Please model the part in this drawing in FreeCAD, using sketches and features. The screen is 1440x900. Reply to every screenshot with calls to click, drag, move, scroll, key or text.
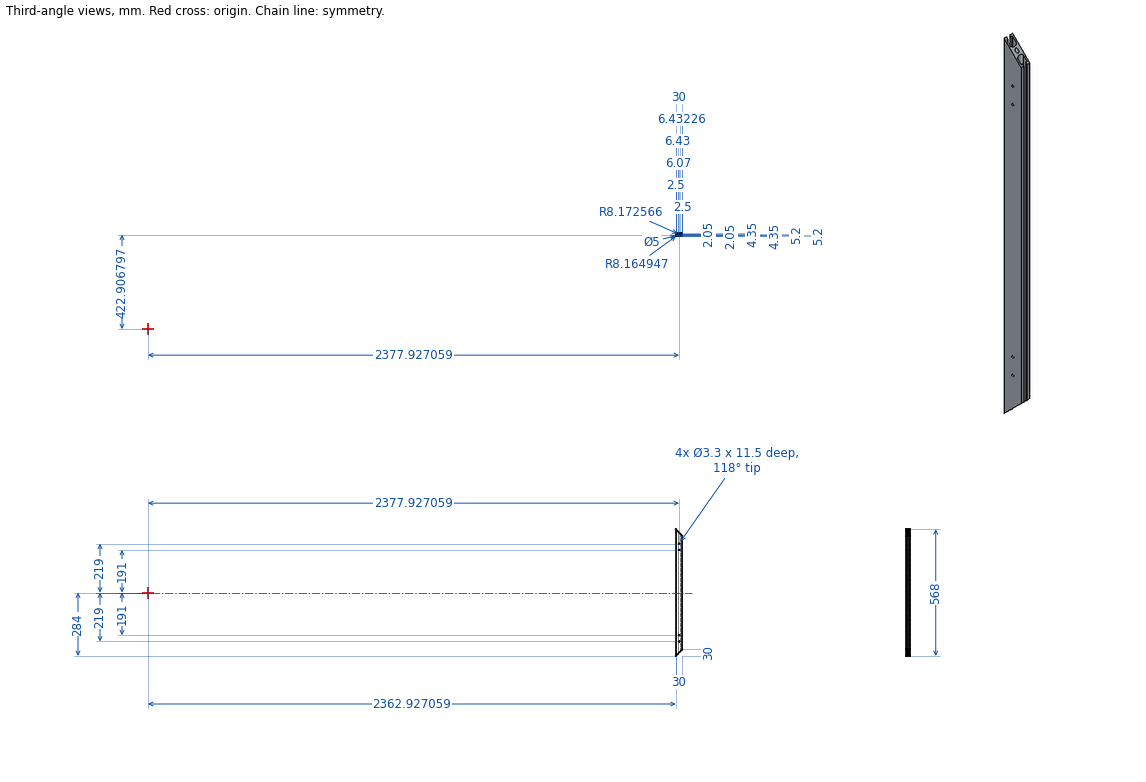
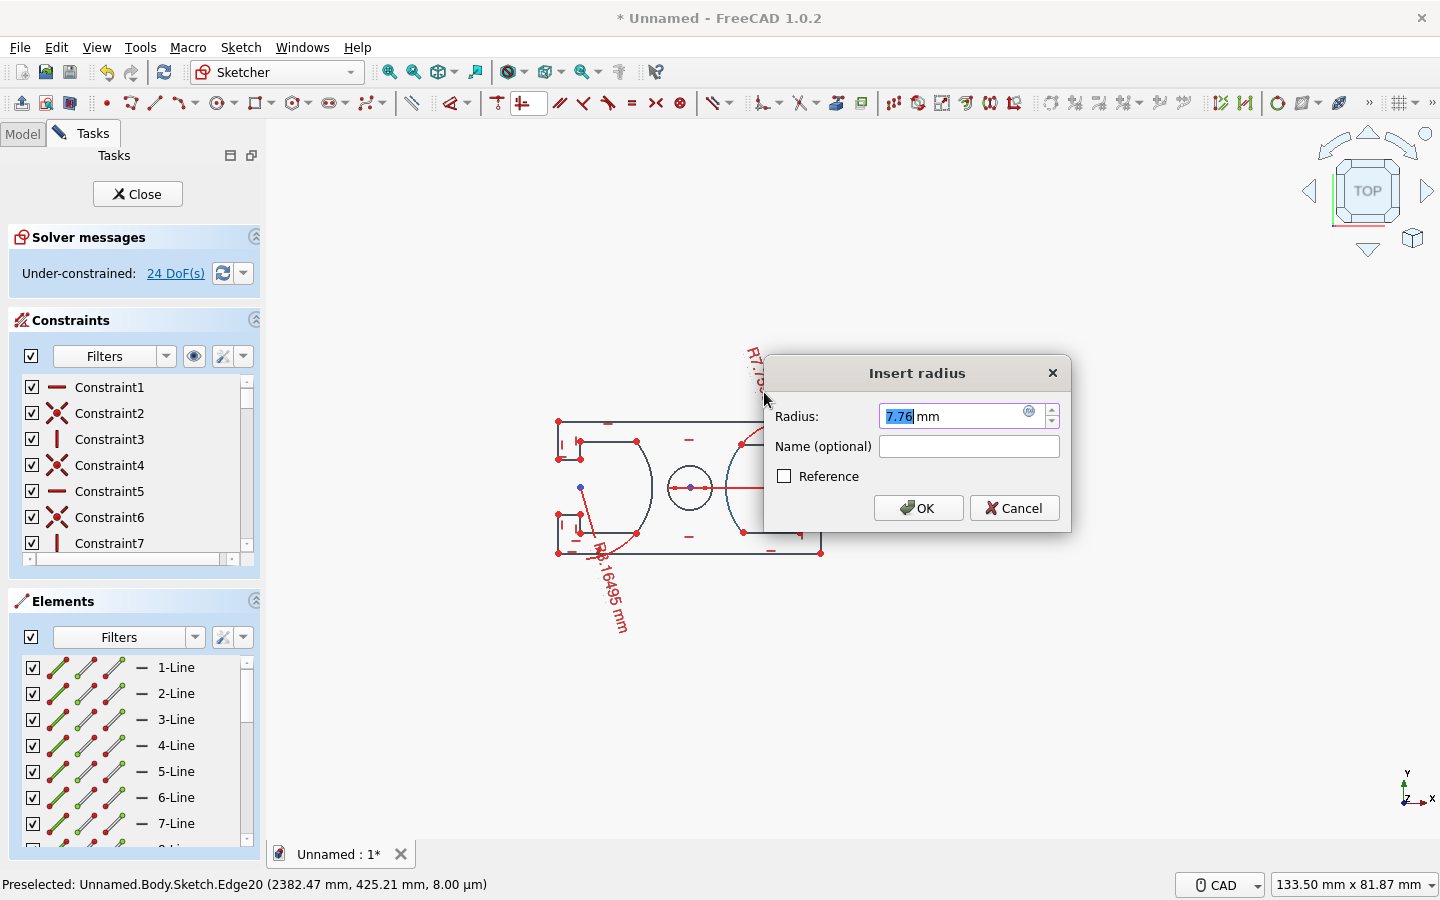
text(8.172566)
key(Return)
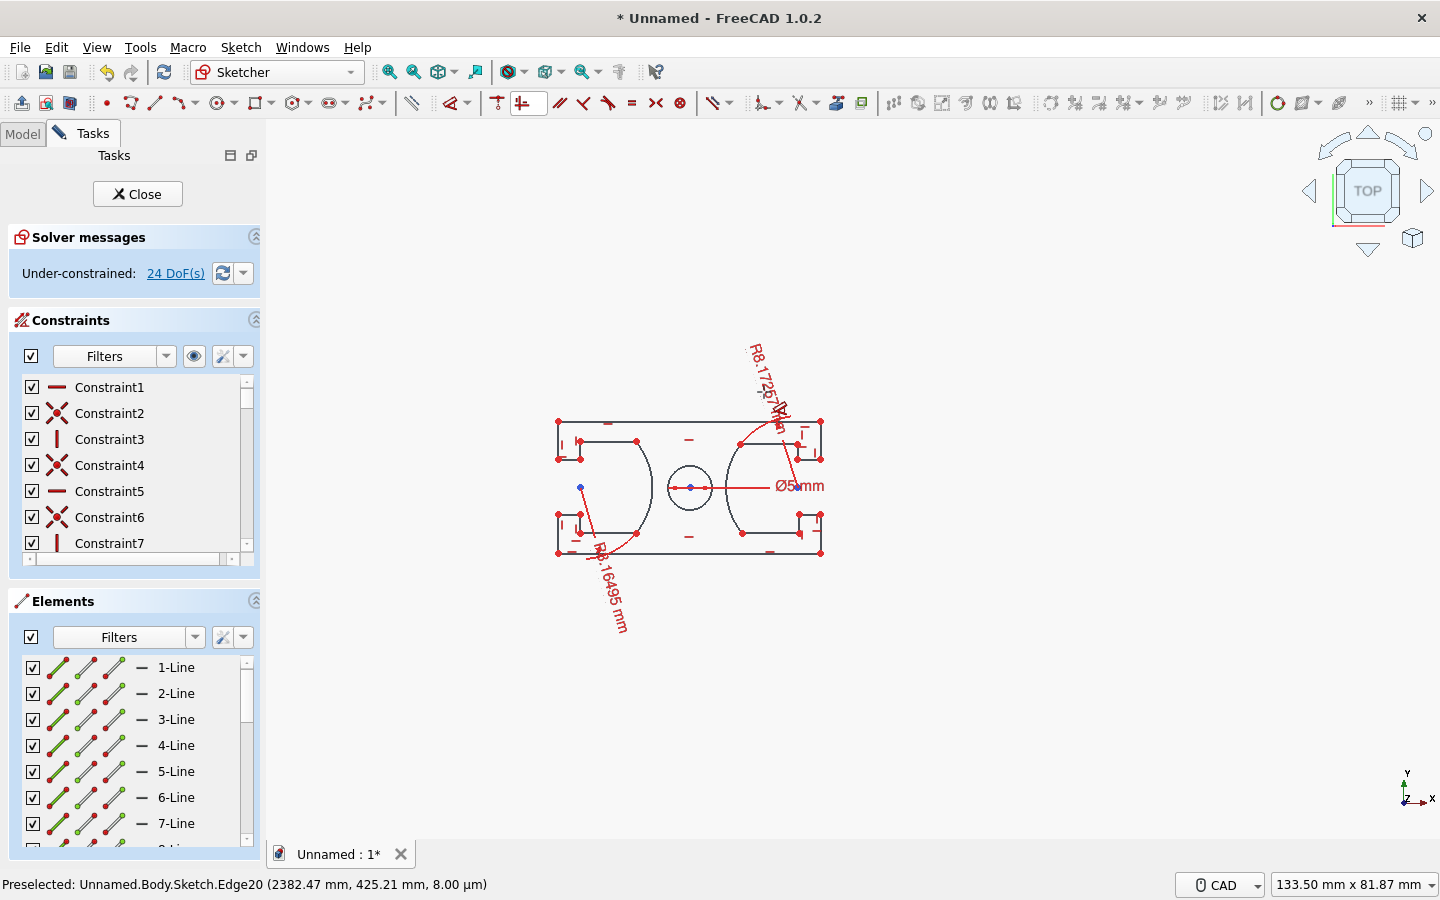
click(742, 422)
click(689, 388)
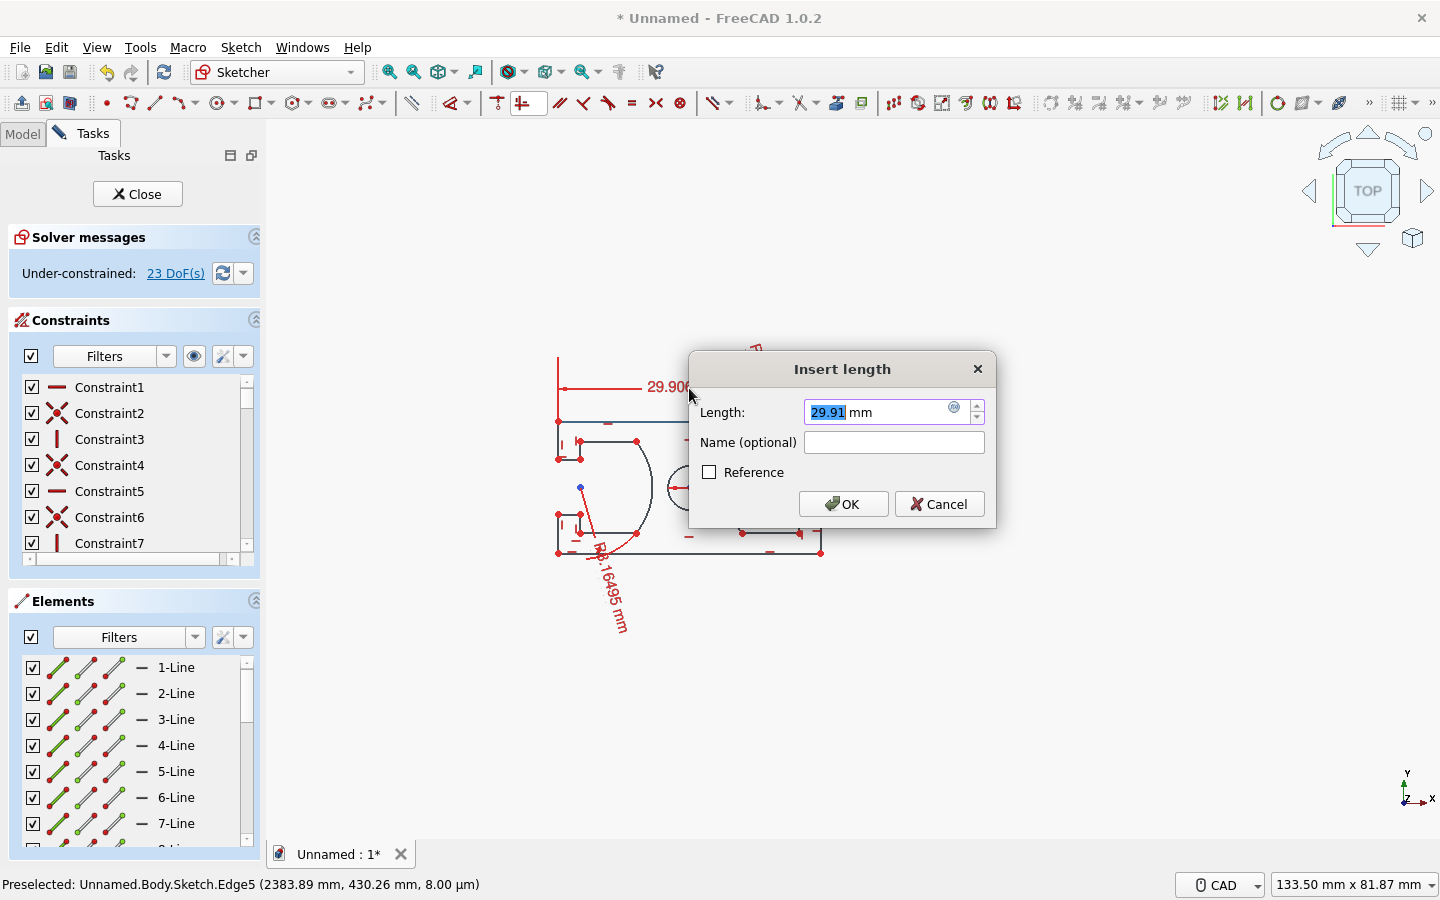
text(30)
key(Return)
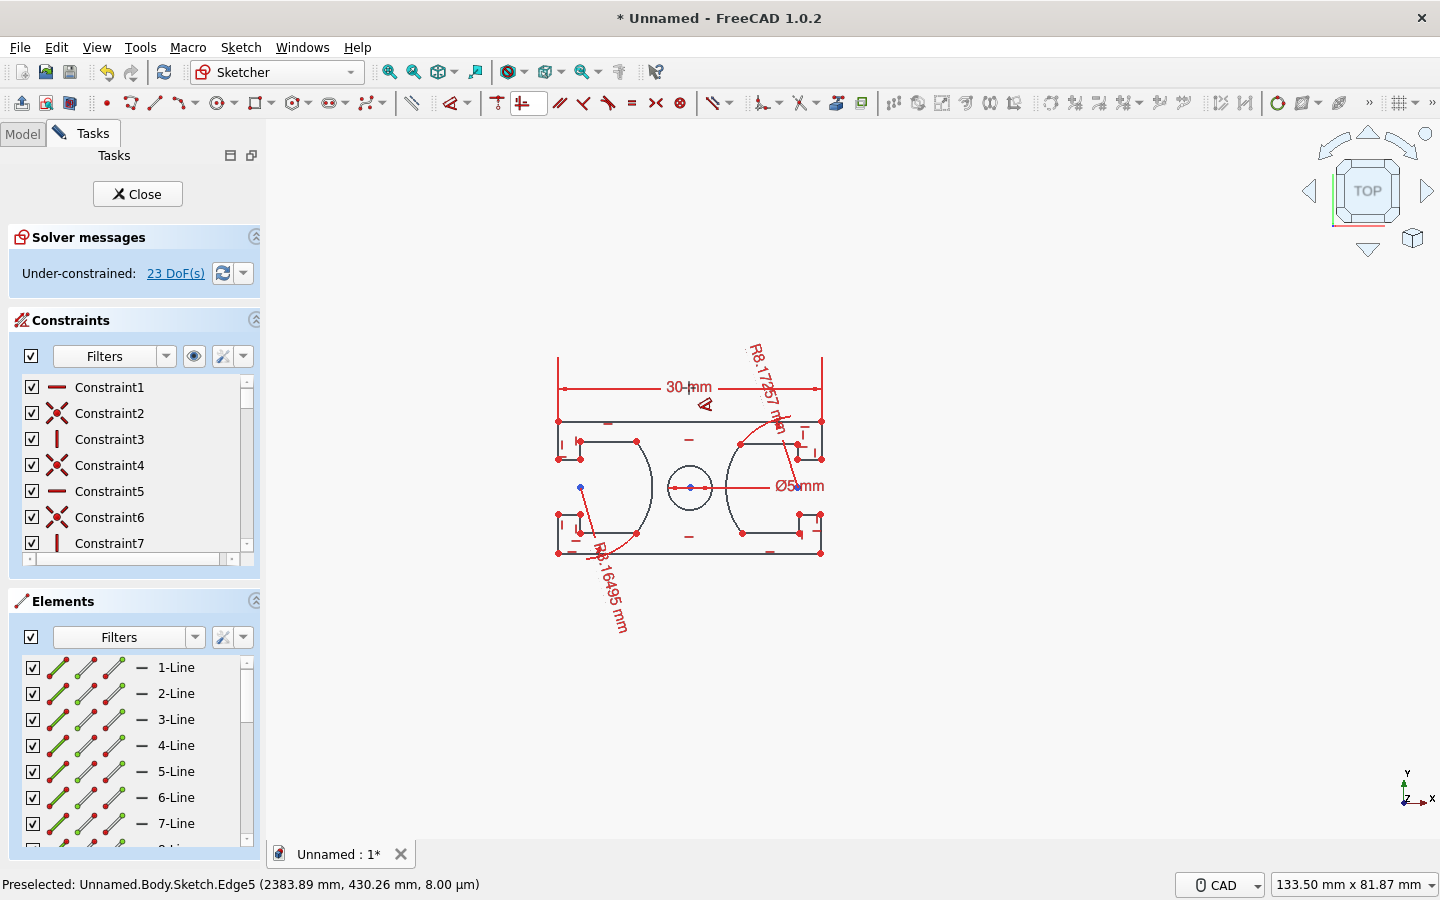
click(637, 554)
click(689, 588)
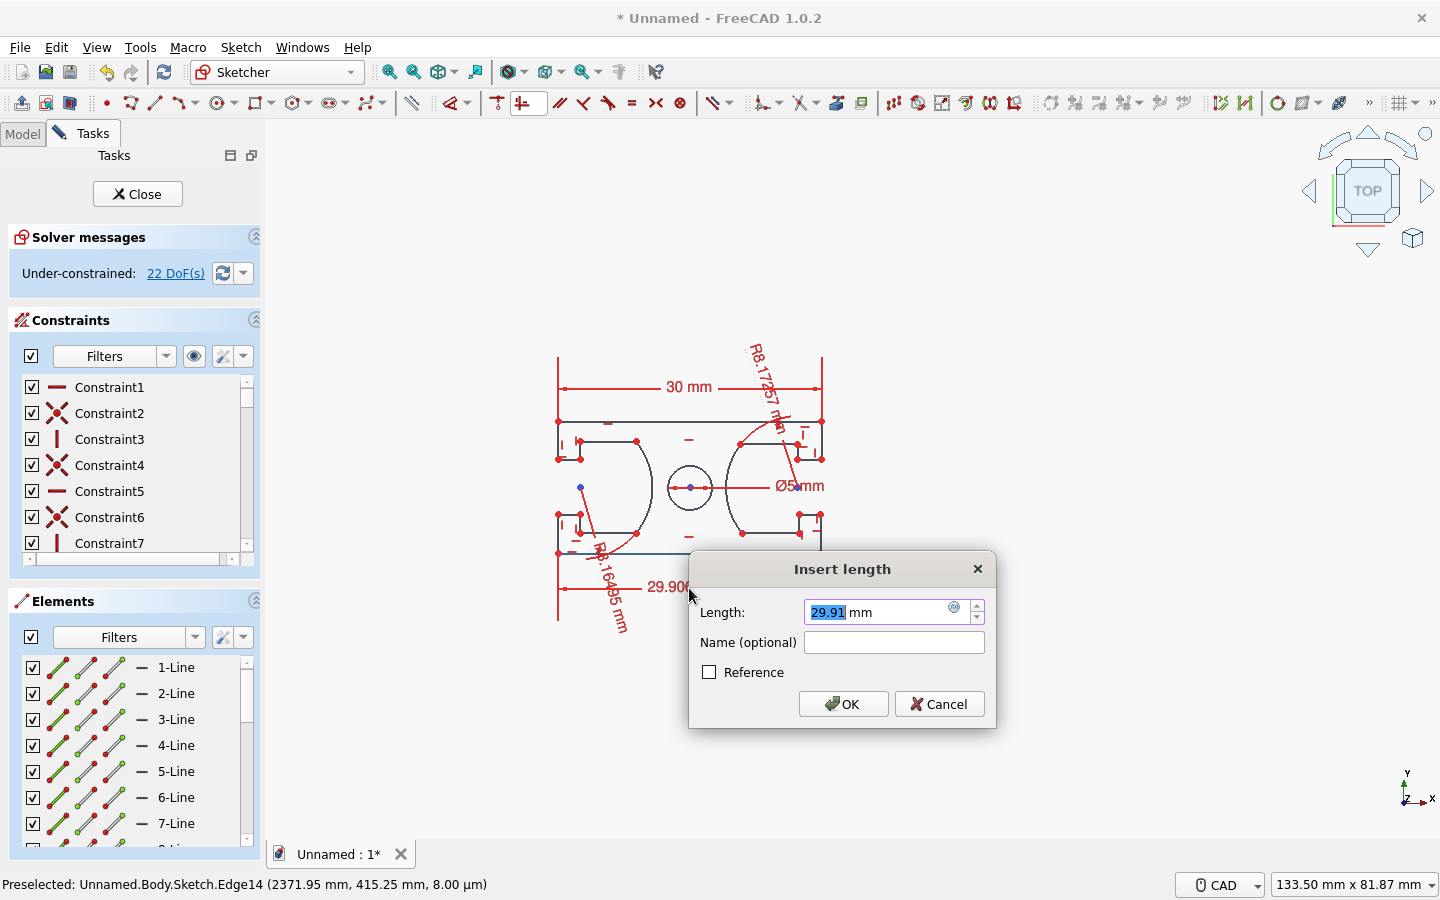
text(30)
key(Return)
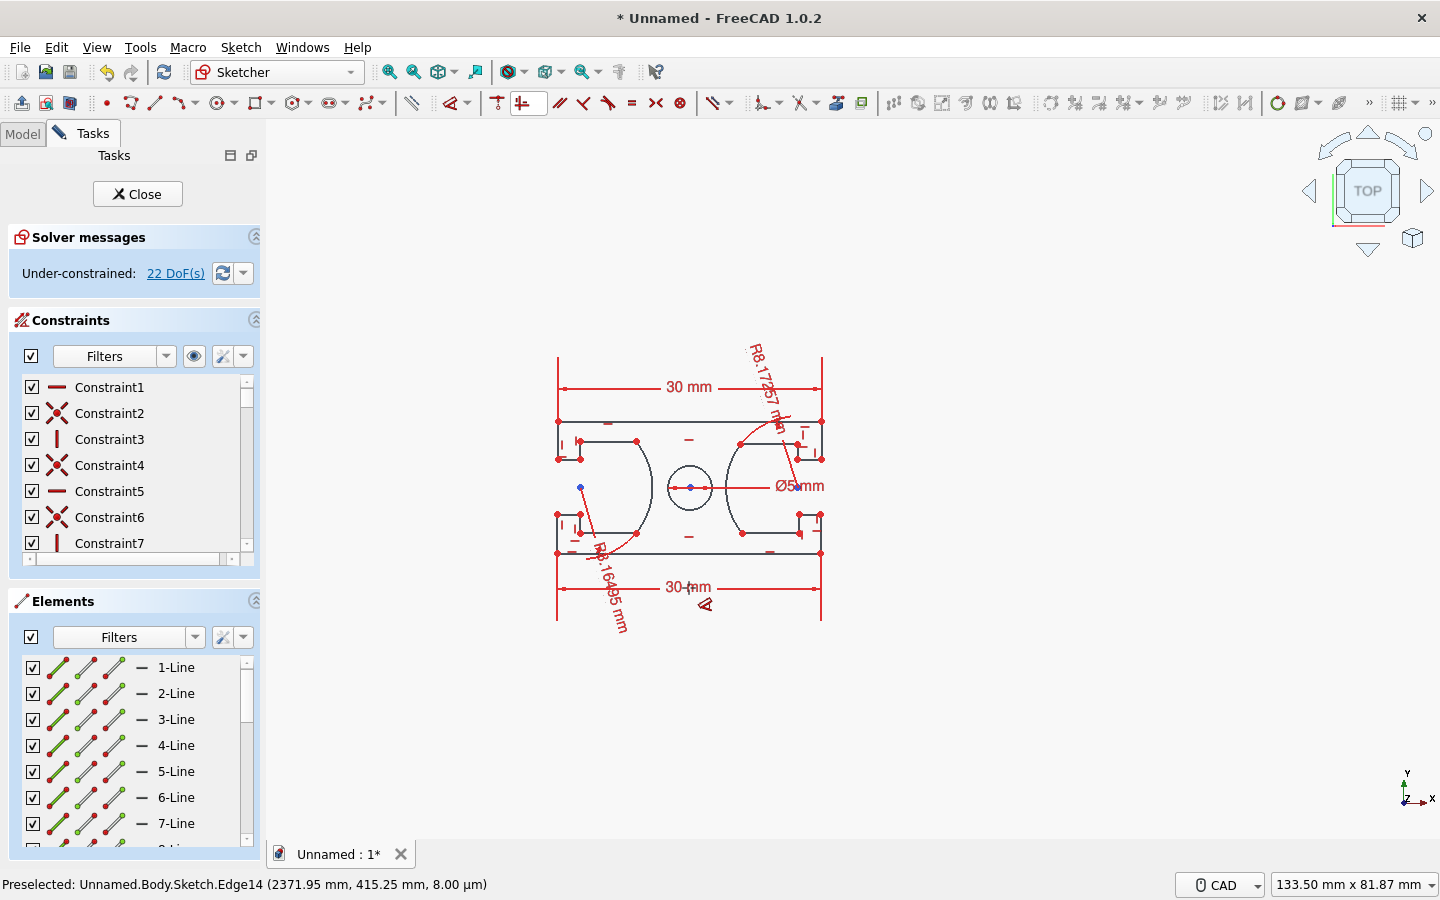
scroll(807, 460, up, 3)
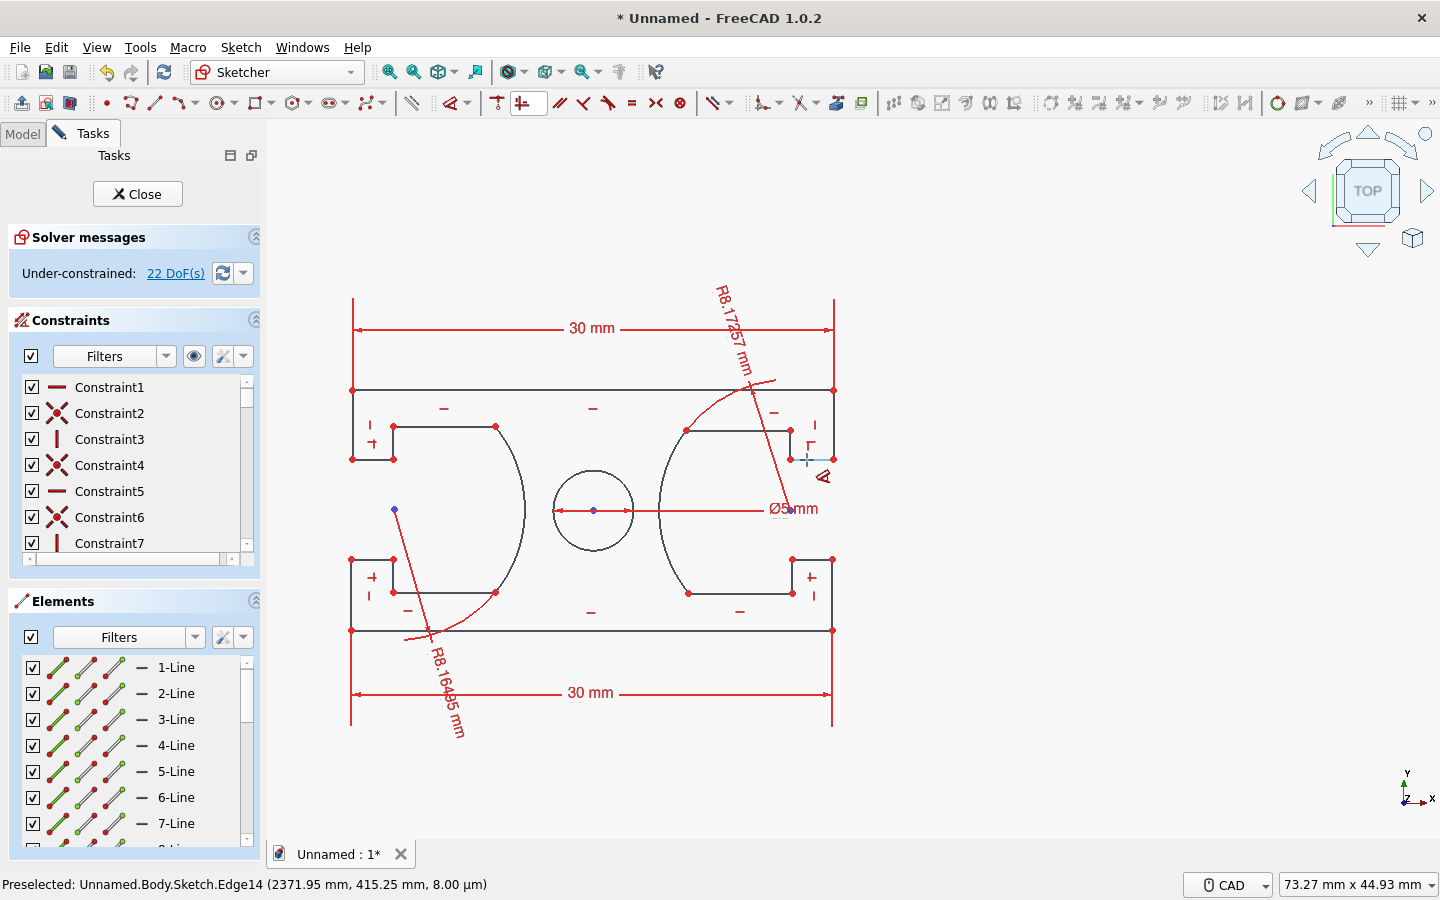
click(808, 460)
click(812, 426)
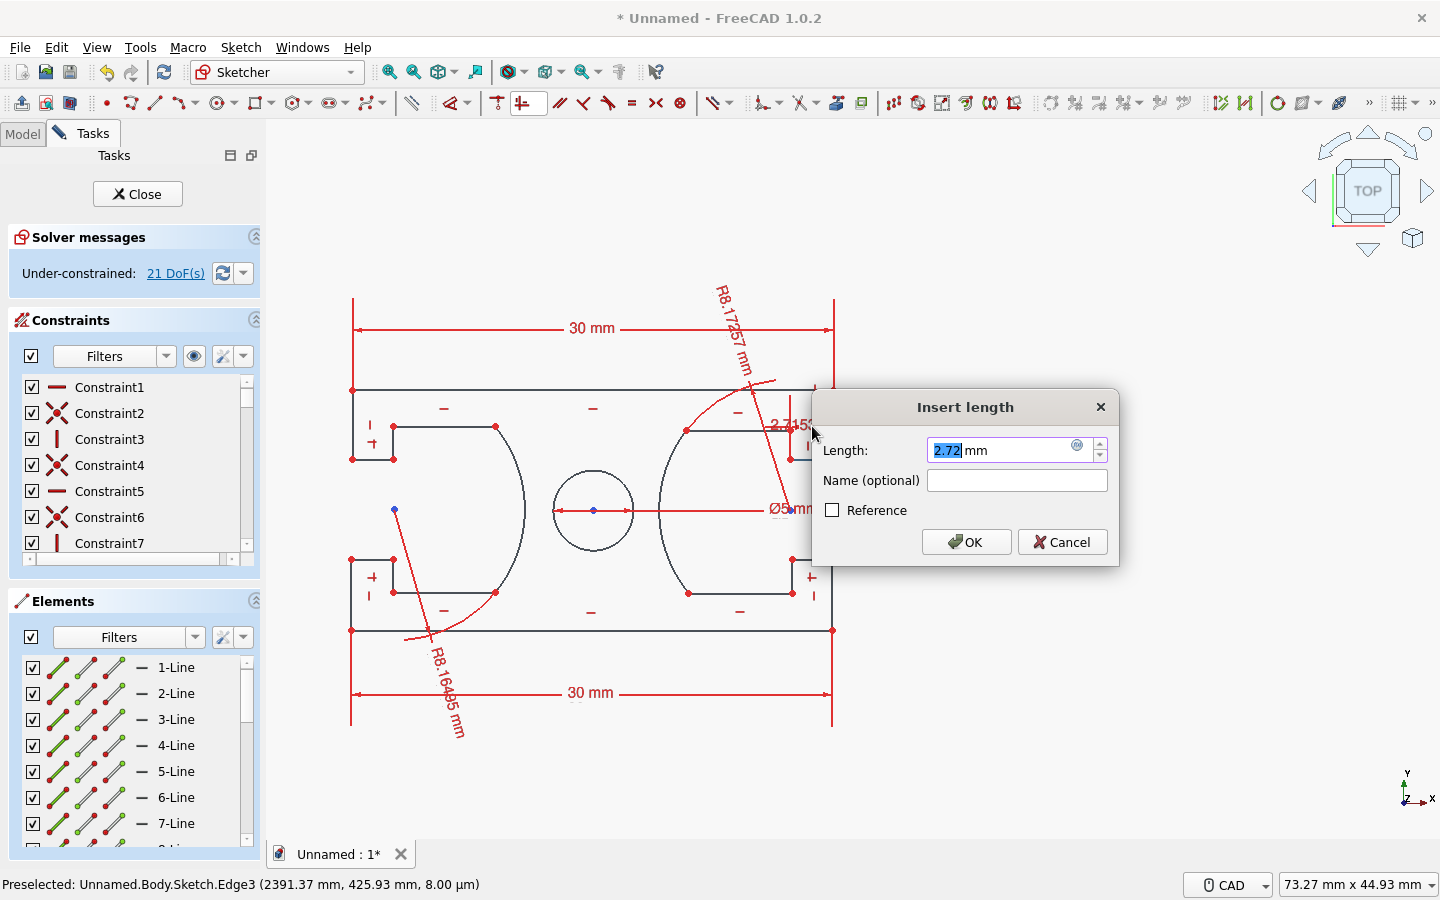
text(2.5)
key(Return)